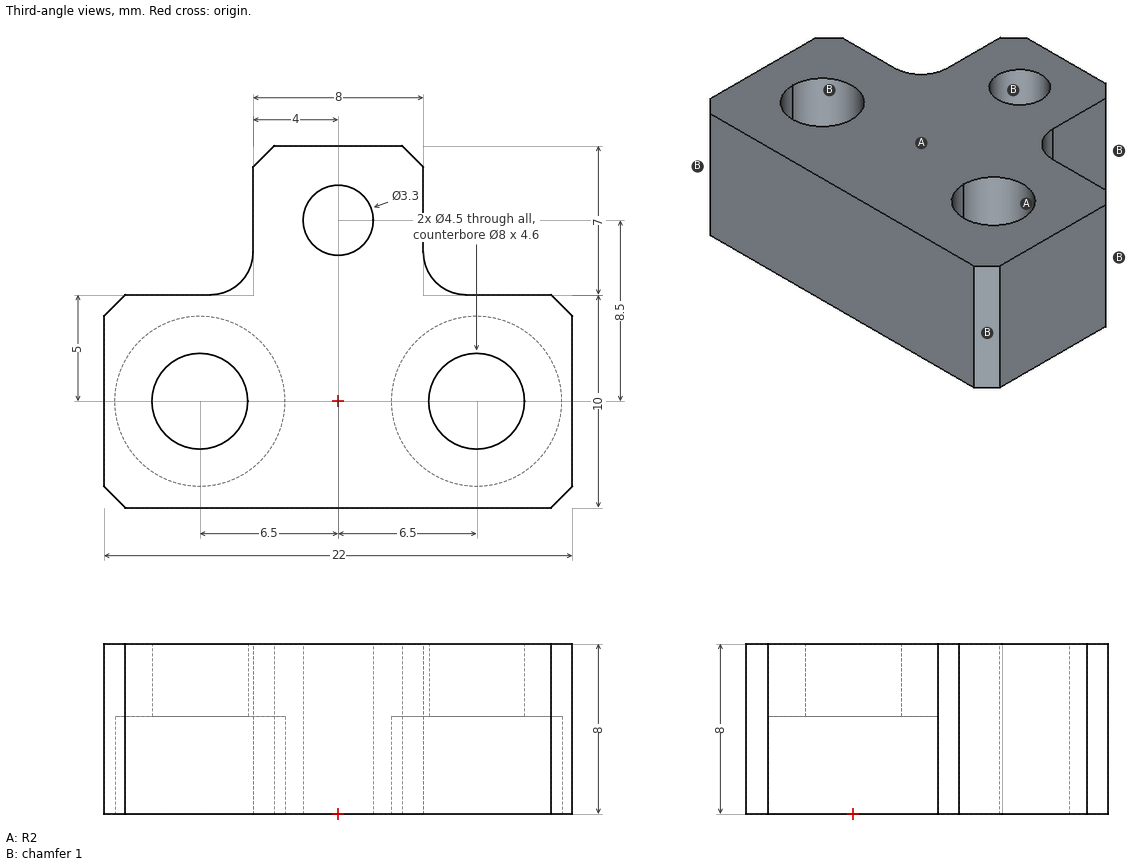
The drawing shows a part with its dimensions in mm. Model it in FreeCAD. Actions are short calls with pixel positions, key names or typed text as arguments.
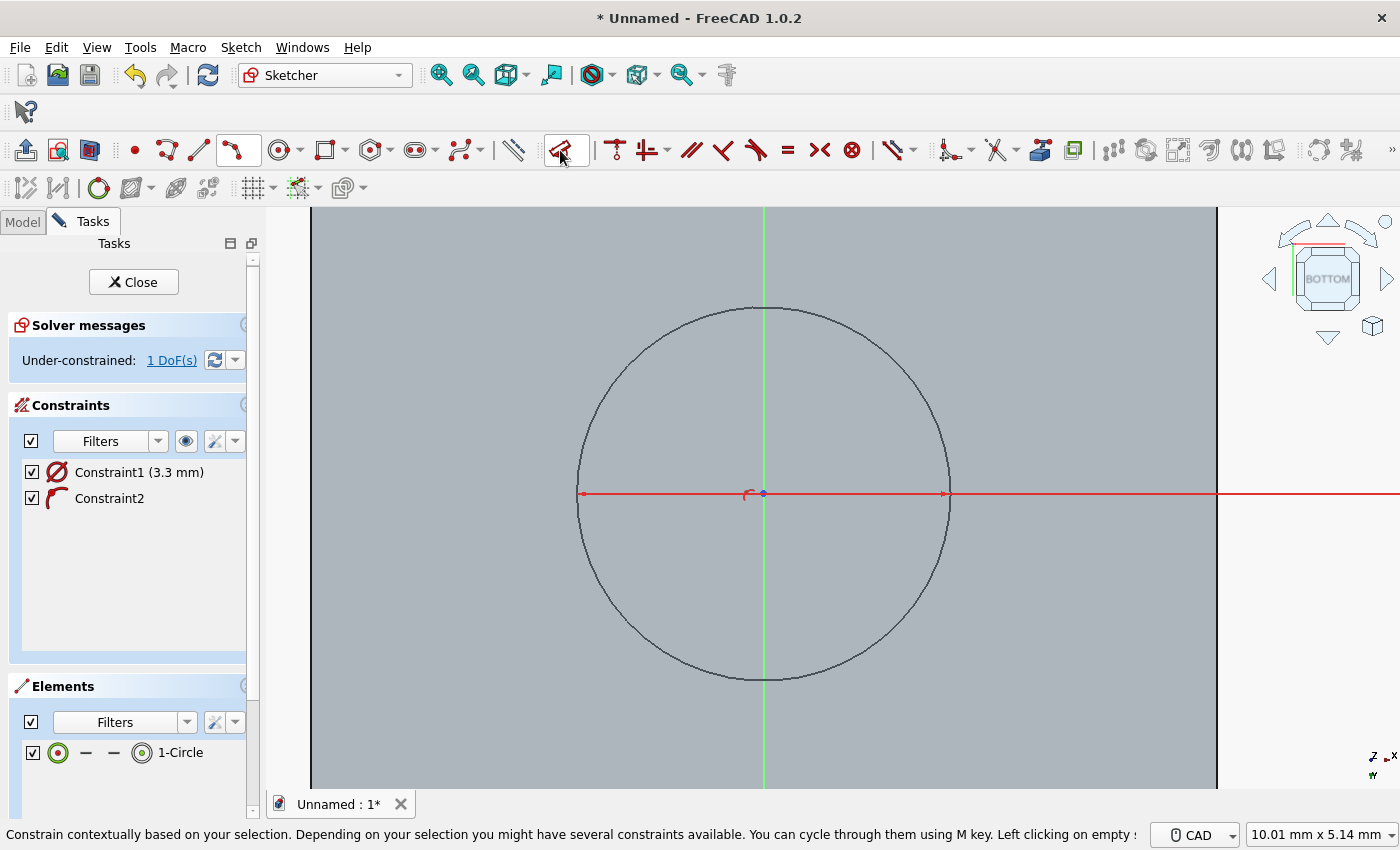
click(764, 494)
click(798, 365)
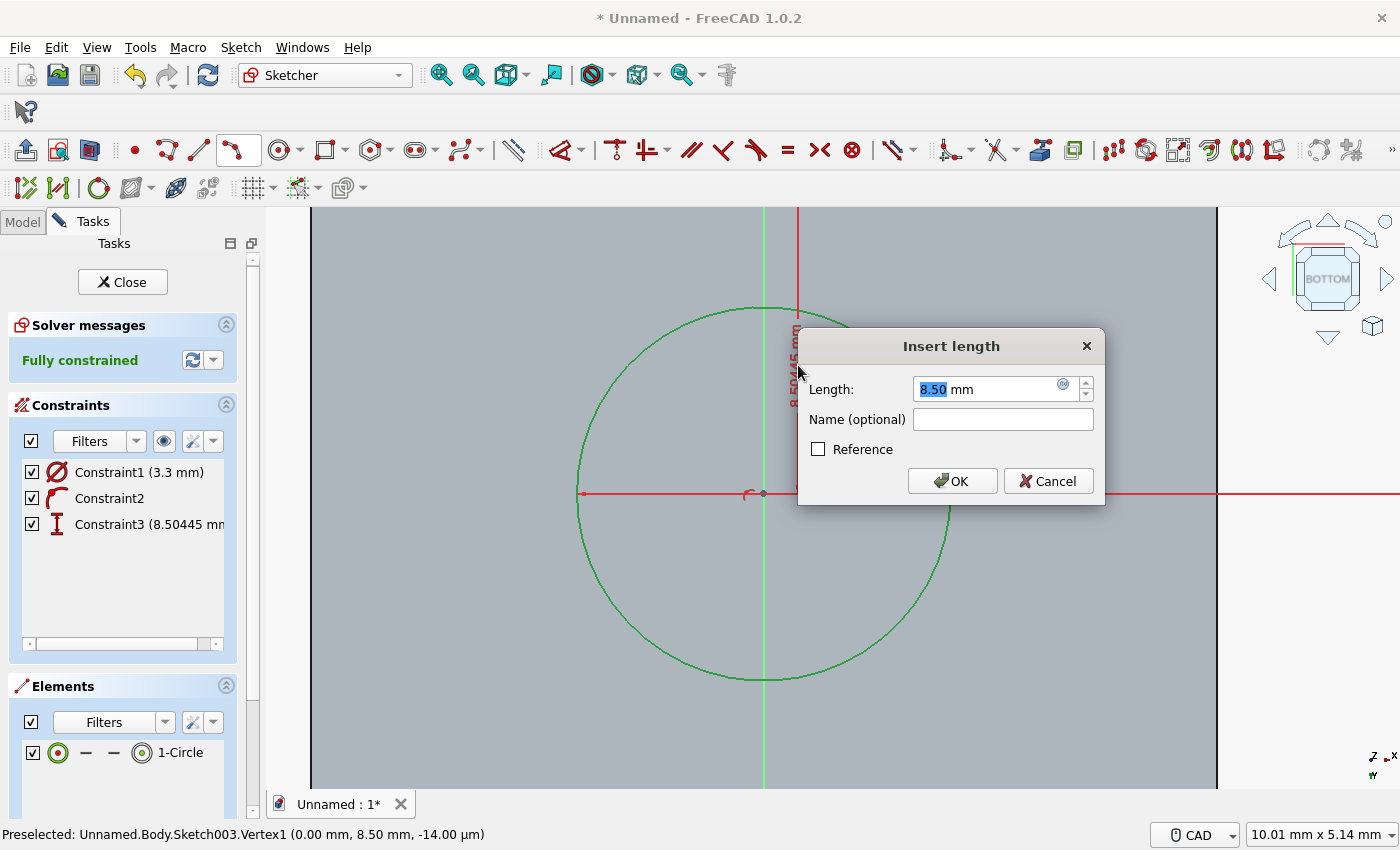
text(8.5)
key(Return)
key(Escape)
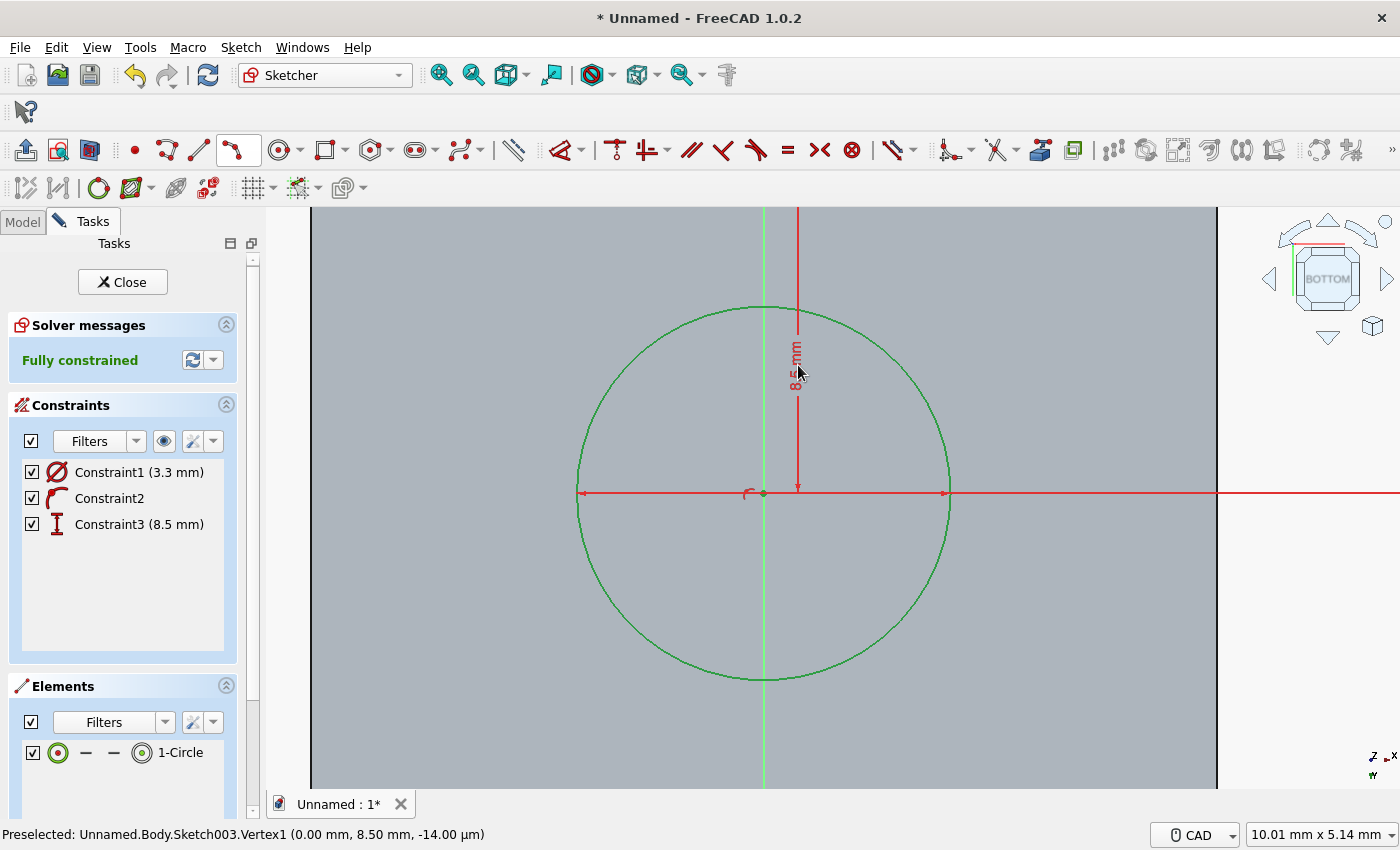
click(123, 282)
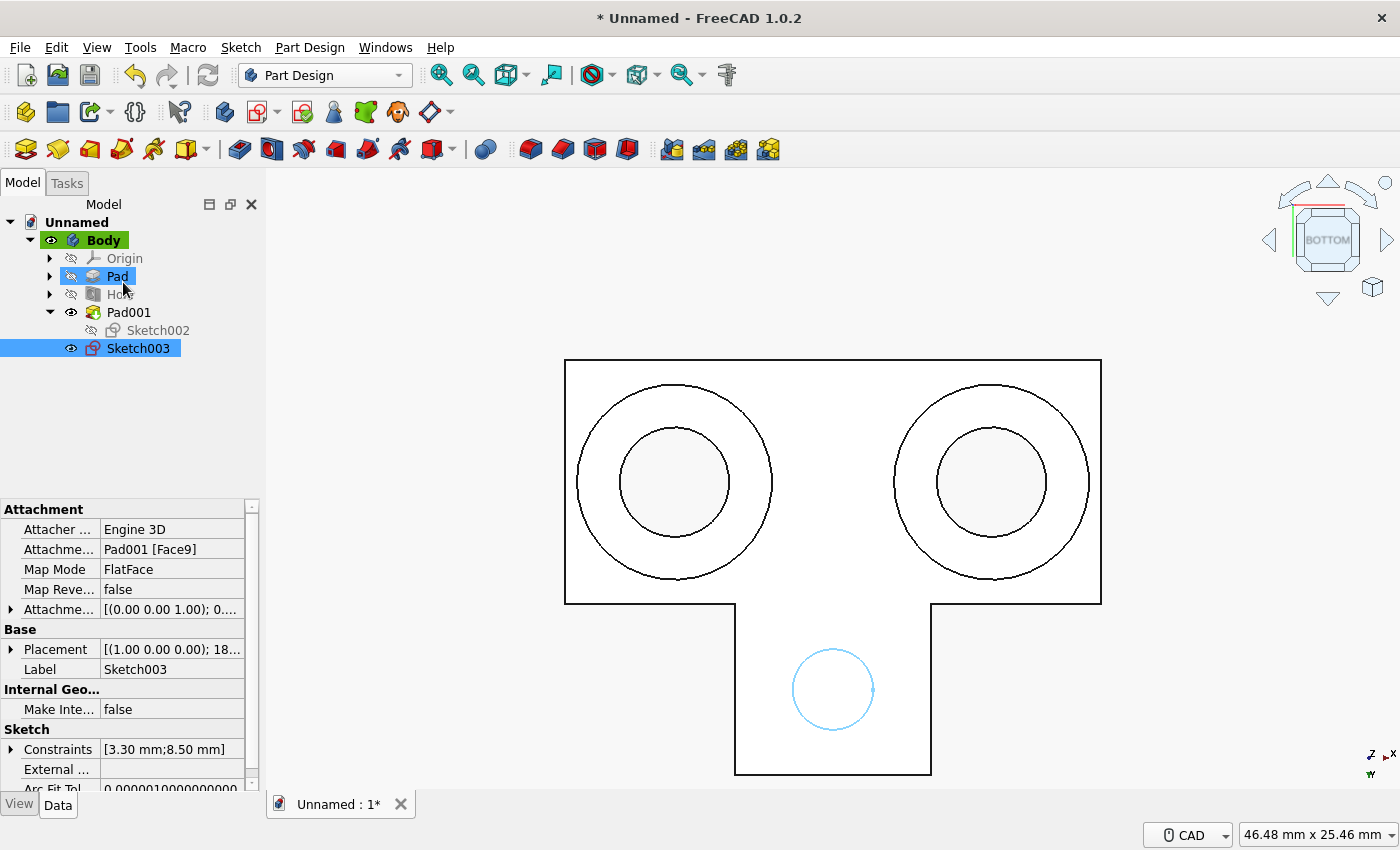
click(240, 150)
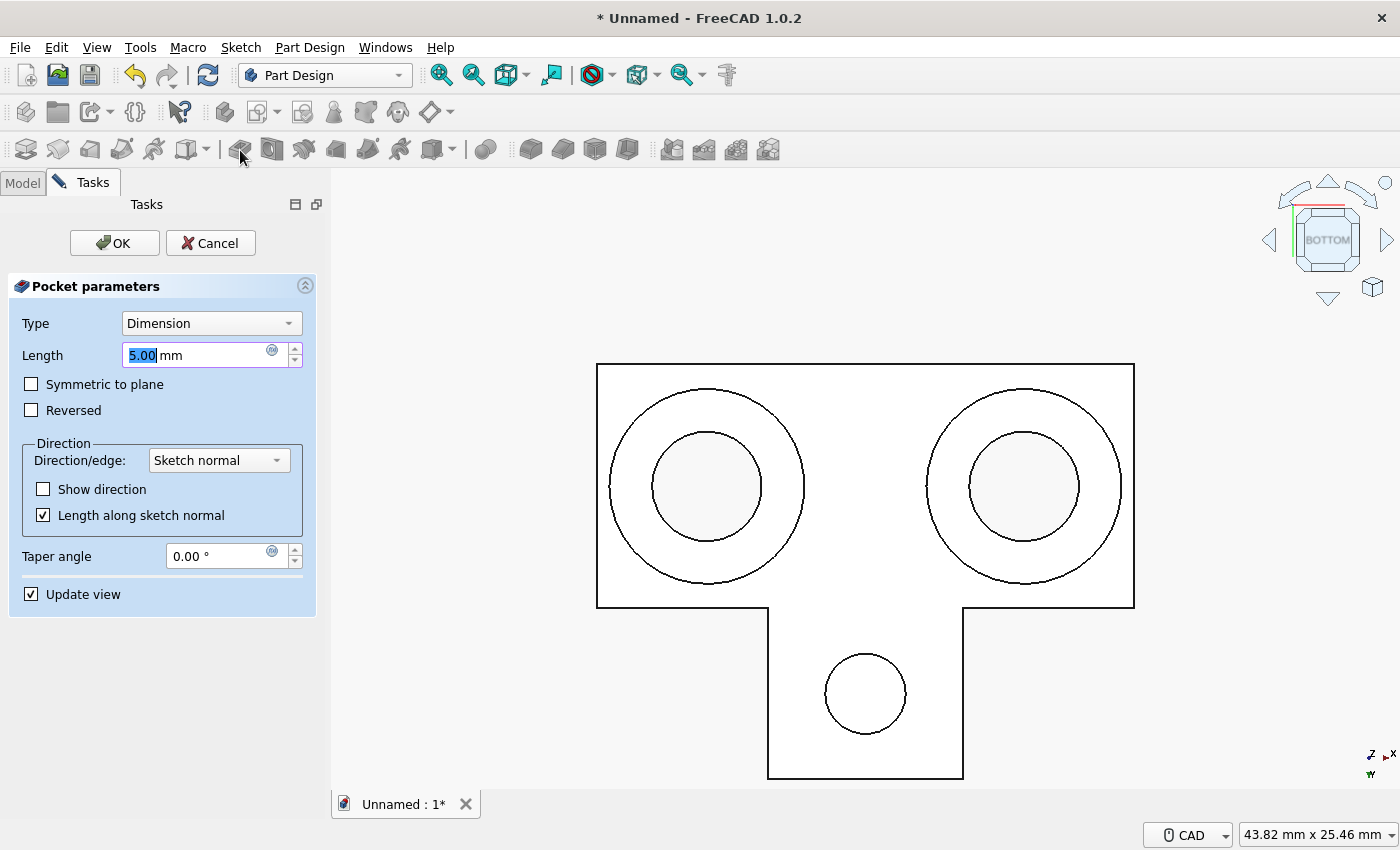
click(212, 324)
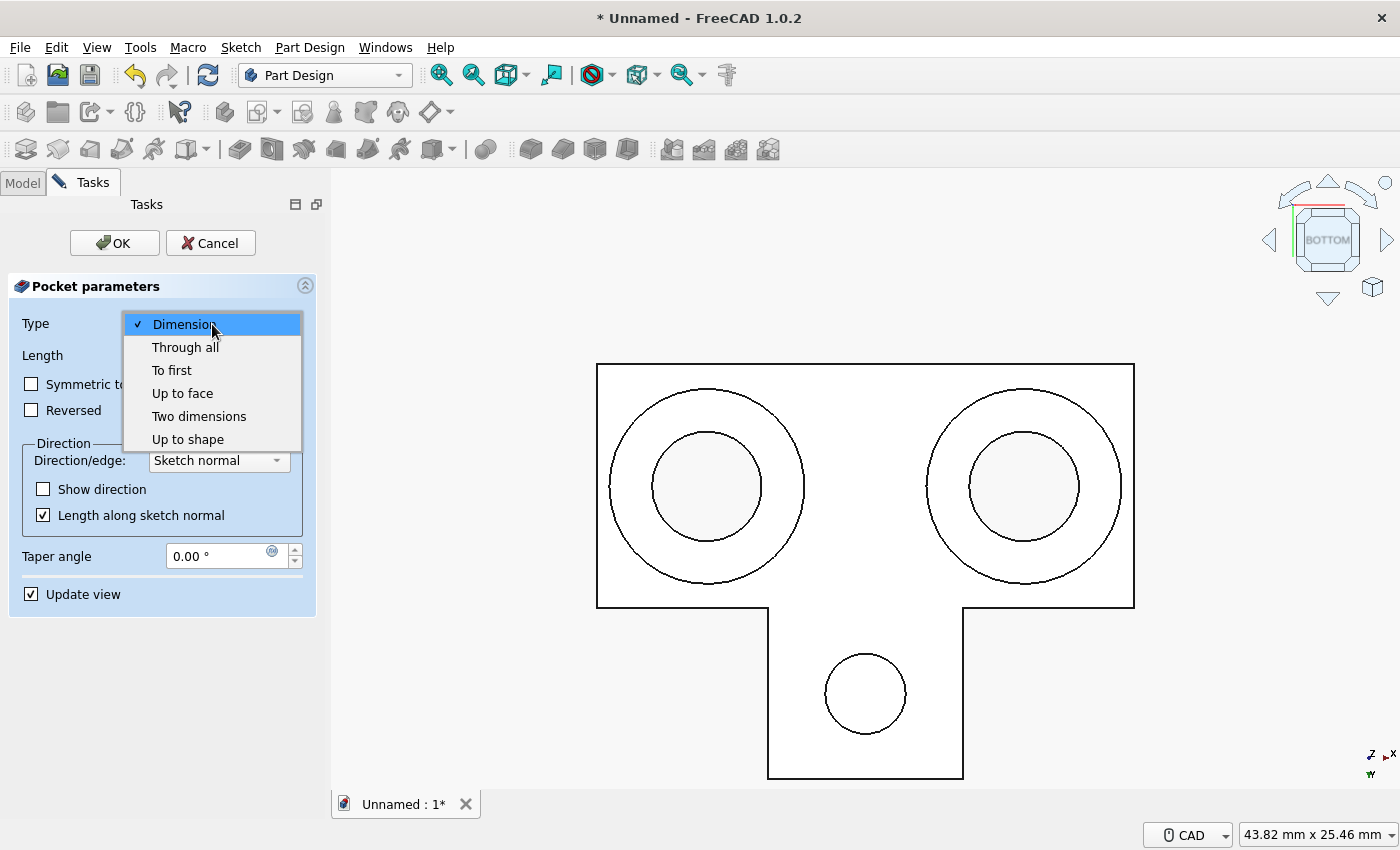
click(212, 348)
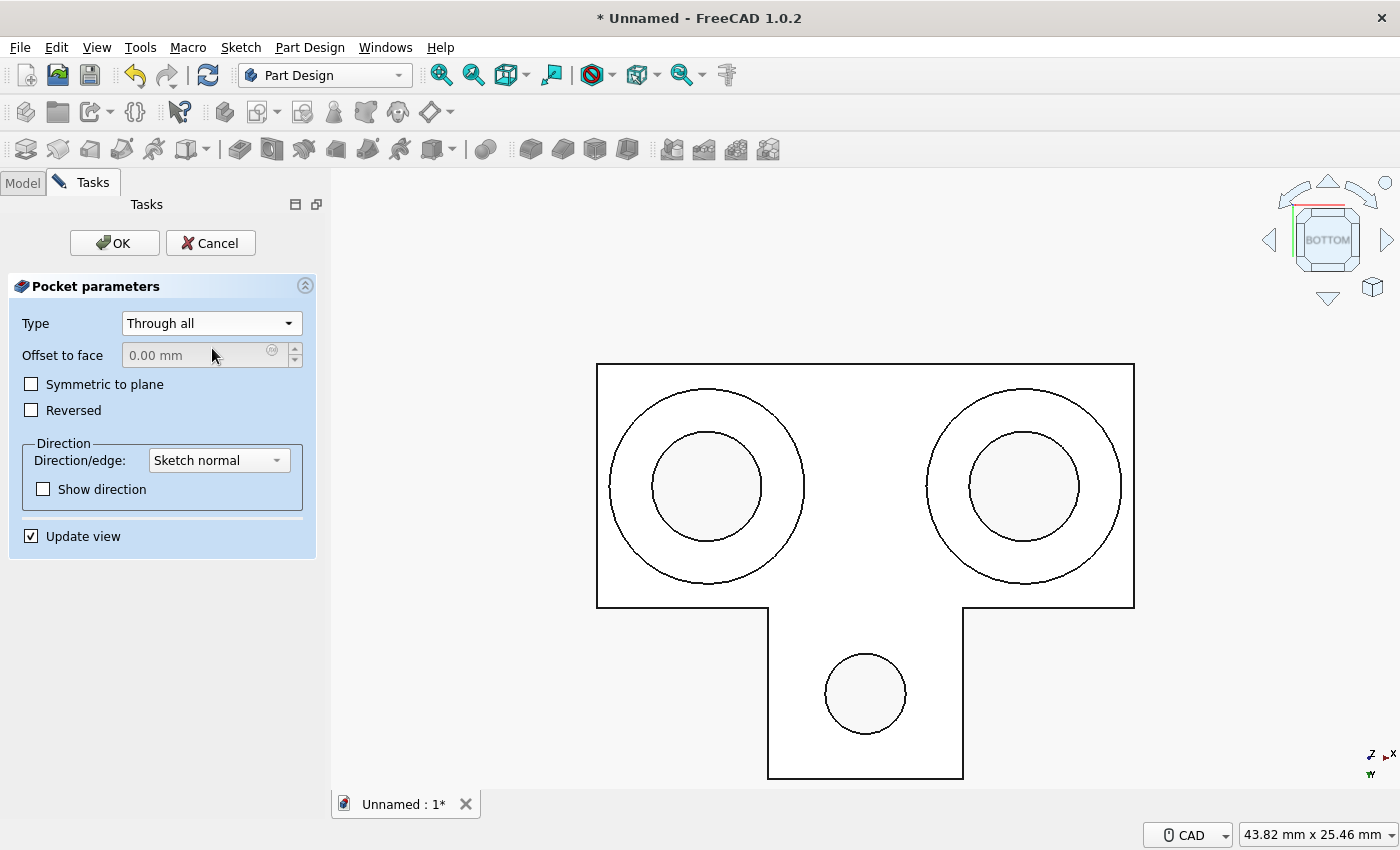
click(115, 243)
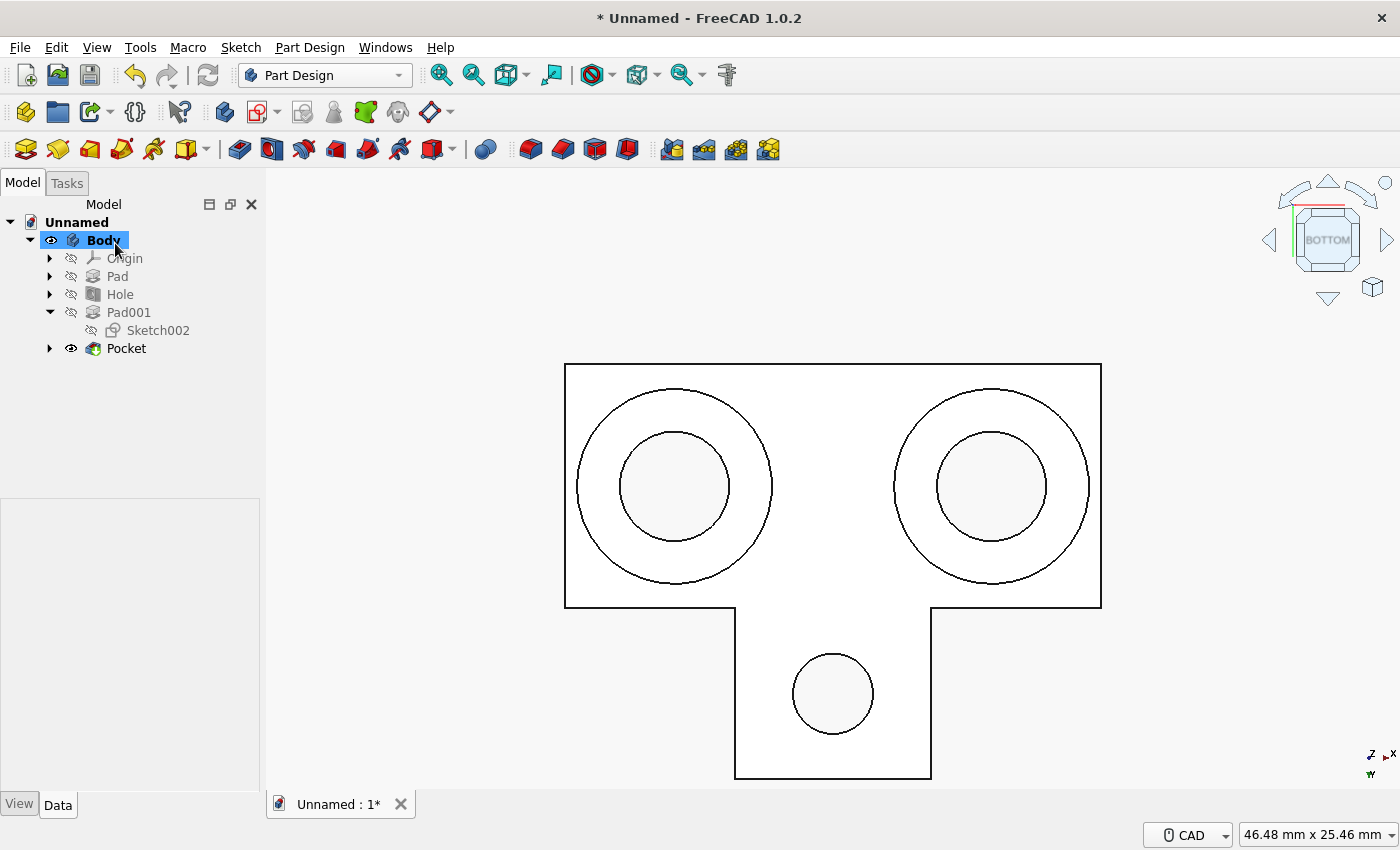
key(0)